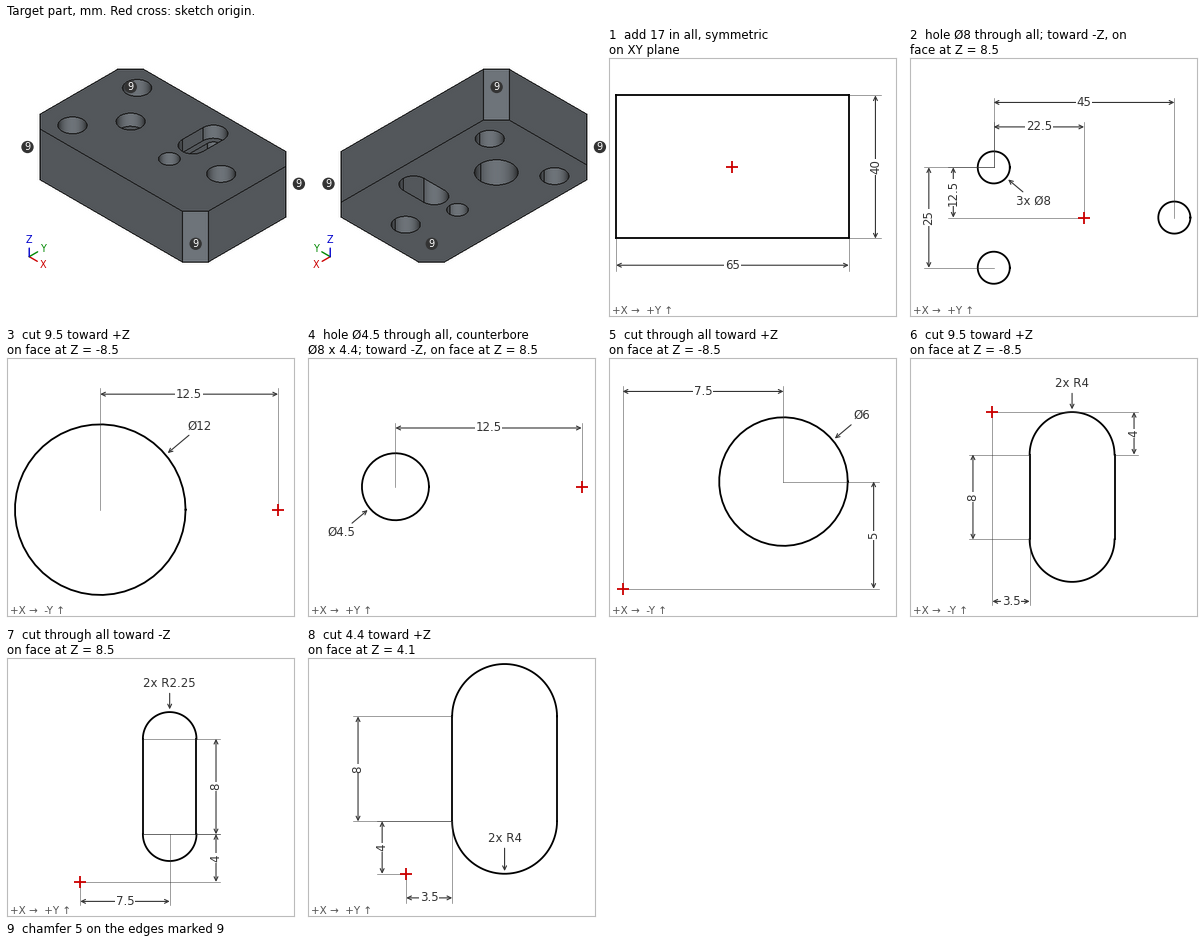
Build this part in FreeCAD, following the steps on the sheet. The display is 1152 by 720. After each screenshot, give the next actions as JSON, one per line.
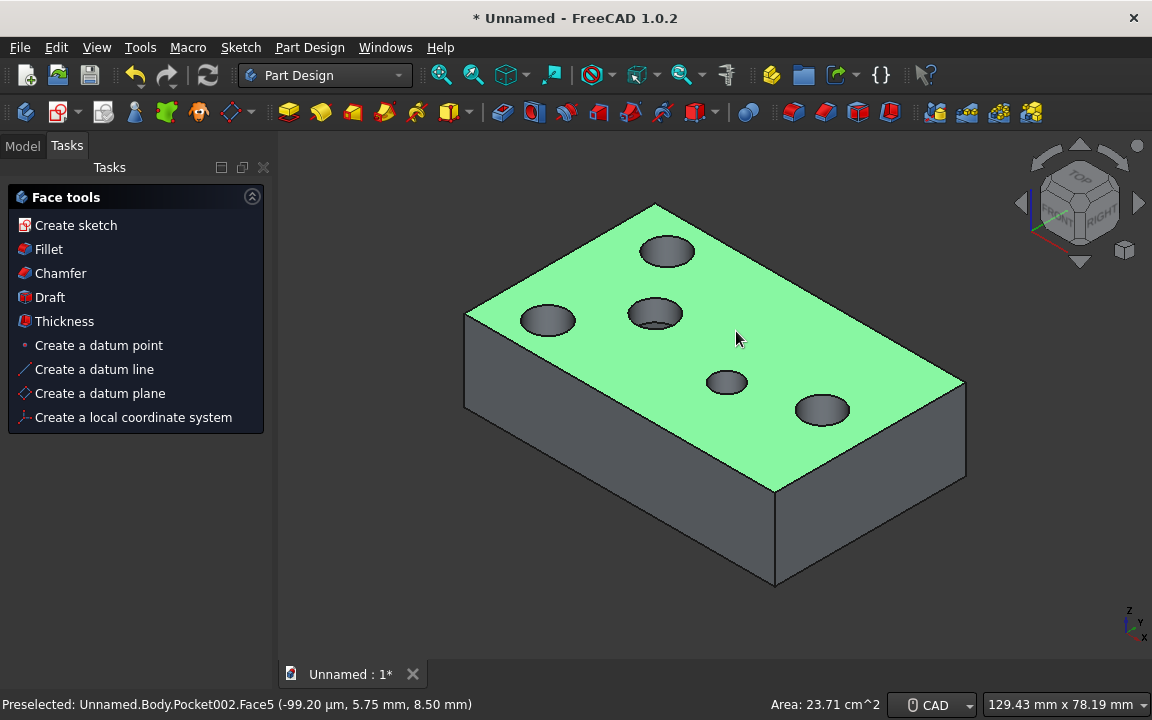
{"action": "left_click", "coordinate": [58, 112]}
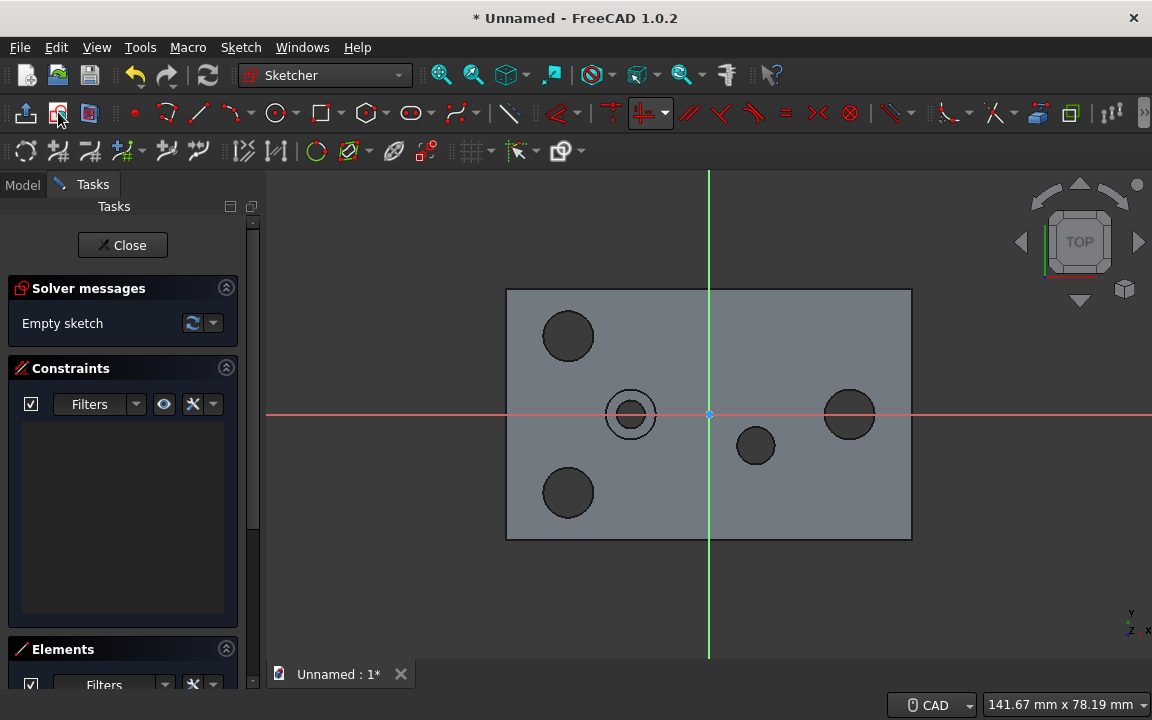
{"action": "scroll", "coordinate": [782, 351], "scroll_direction": "up", "scroll_amount": 6}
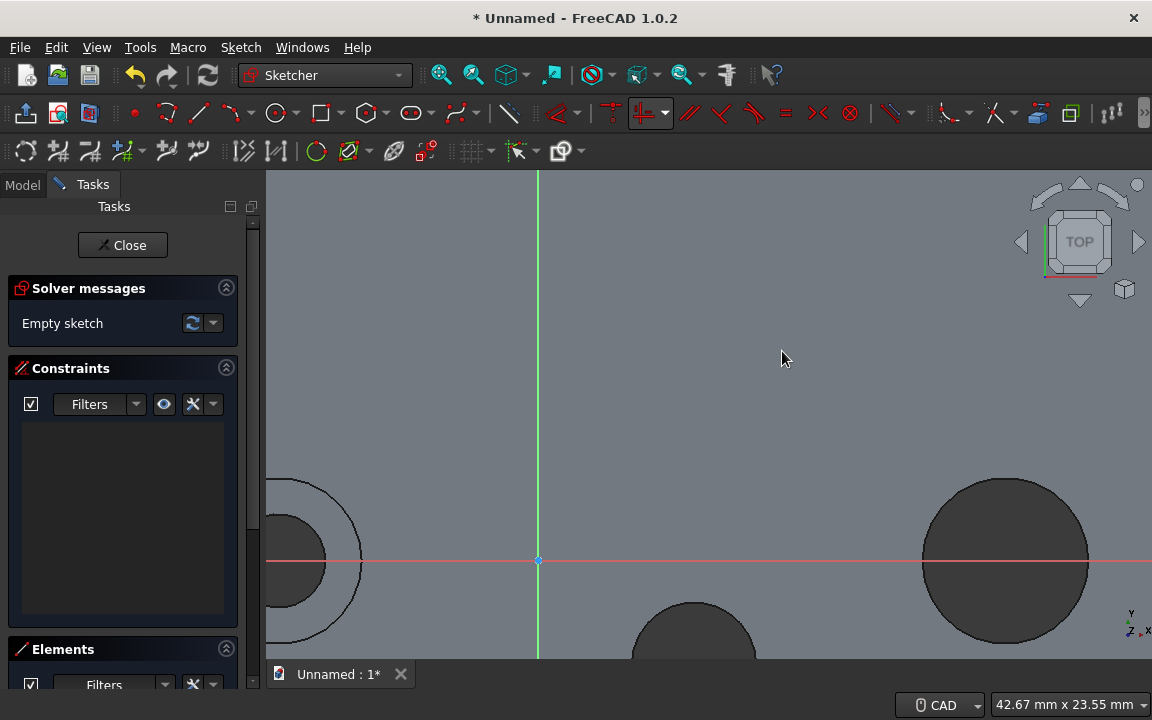
{"action": "key", "text": "g s"}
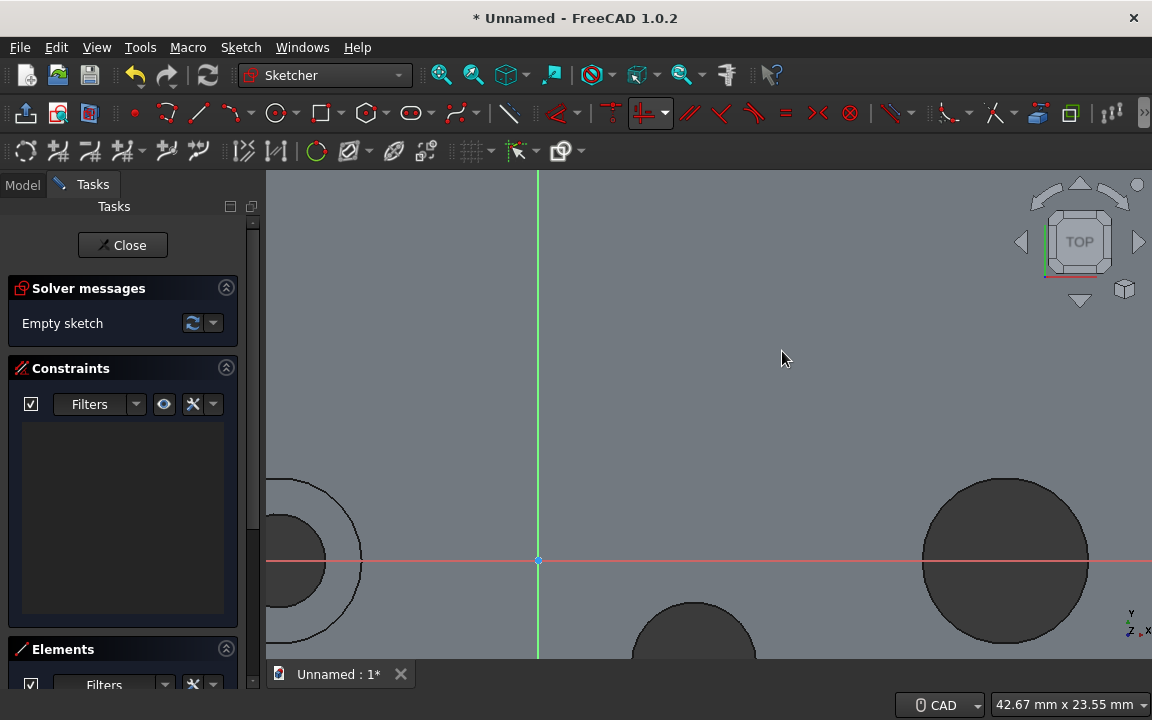
{"action": "left_click", "coordinate": [694, 478]}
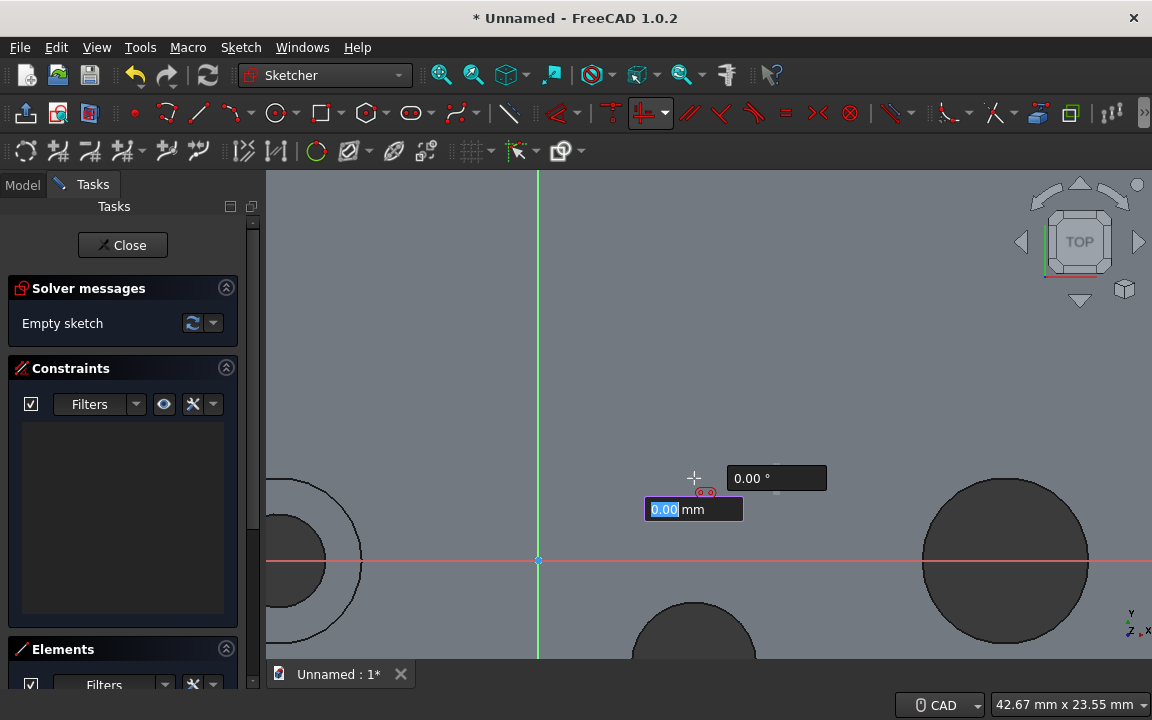
{"action": "left_click", "coordinate": [694, 312]}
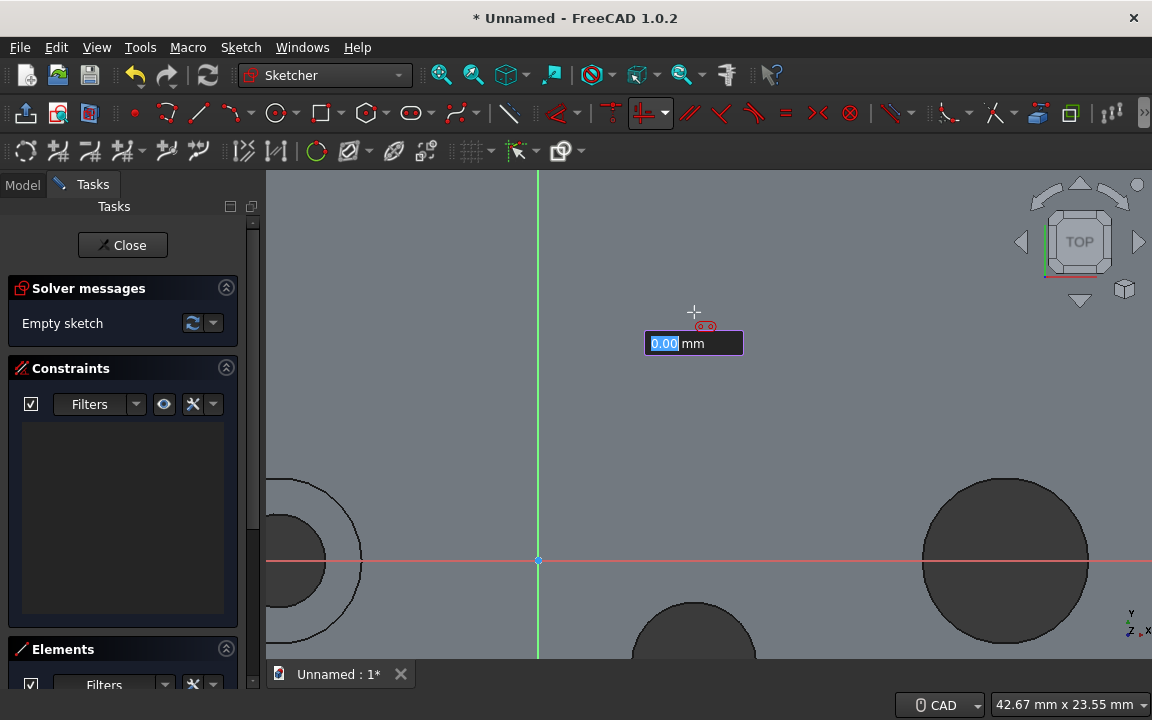
{"action": "left_click", "coordinate": [647, 395]}
{"action": "key", "text": "Escape"}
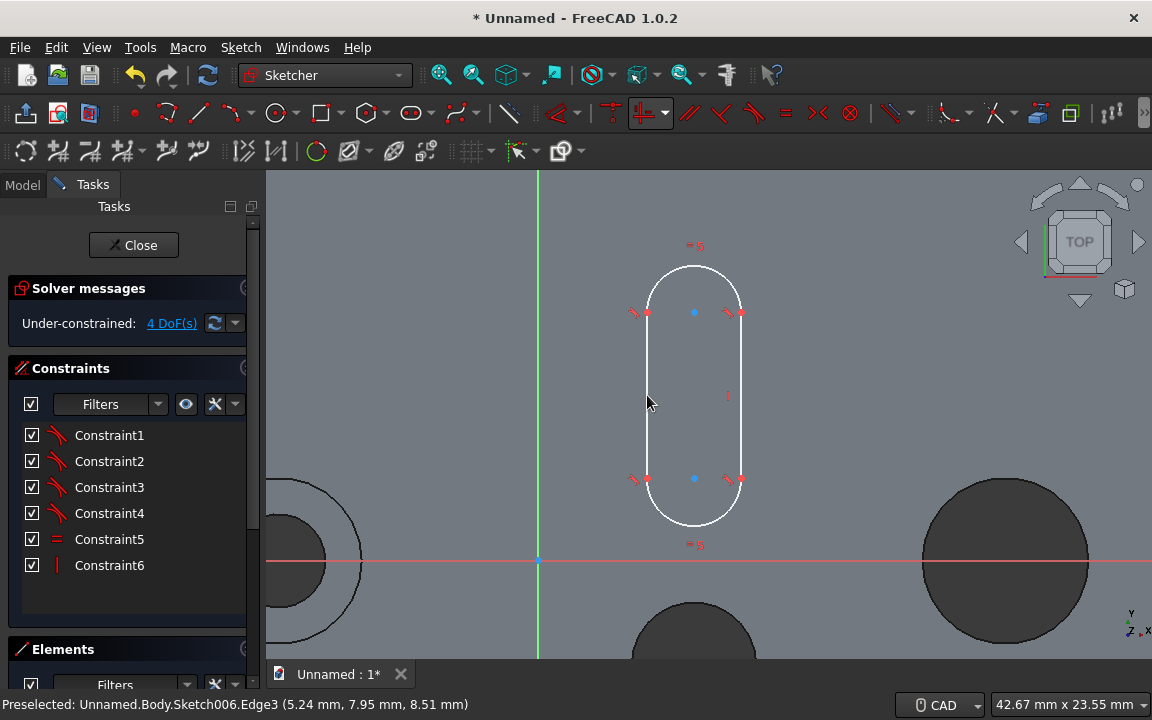
{"action": "left_click", "coordinate": [556, 114]}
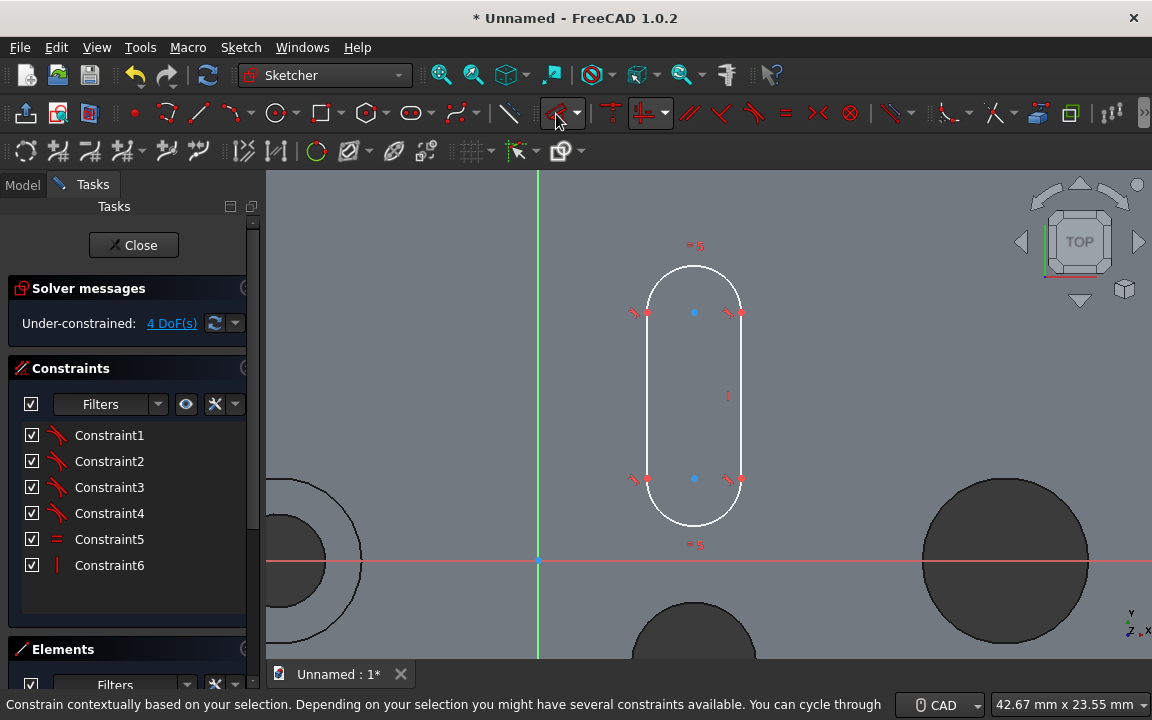
{"action": "left_click", "coordinate": [666, 517]}
{"action": "left_click", "coordinate": [647, 543]}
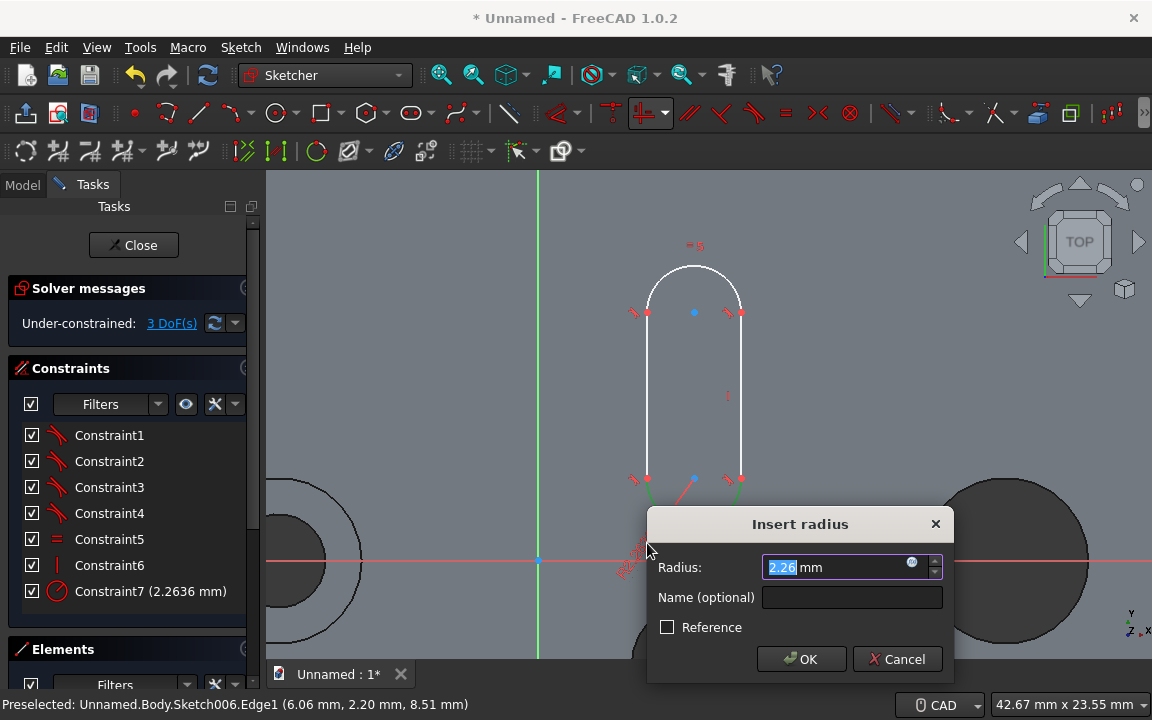
{"action": "type", "text": "2.25"}
{"action": "key", "text": "Return"}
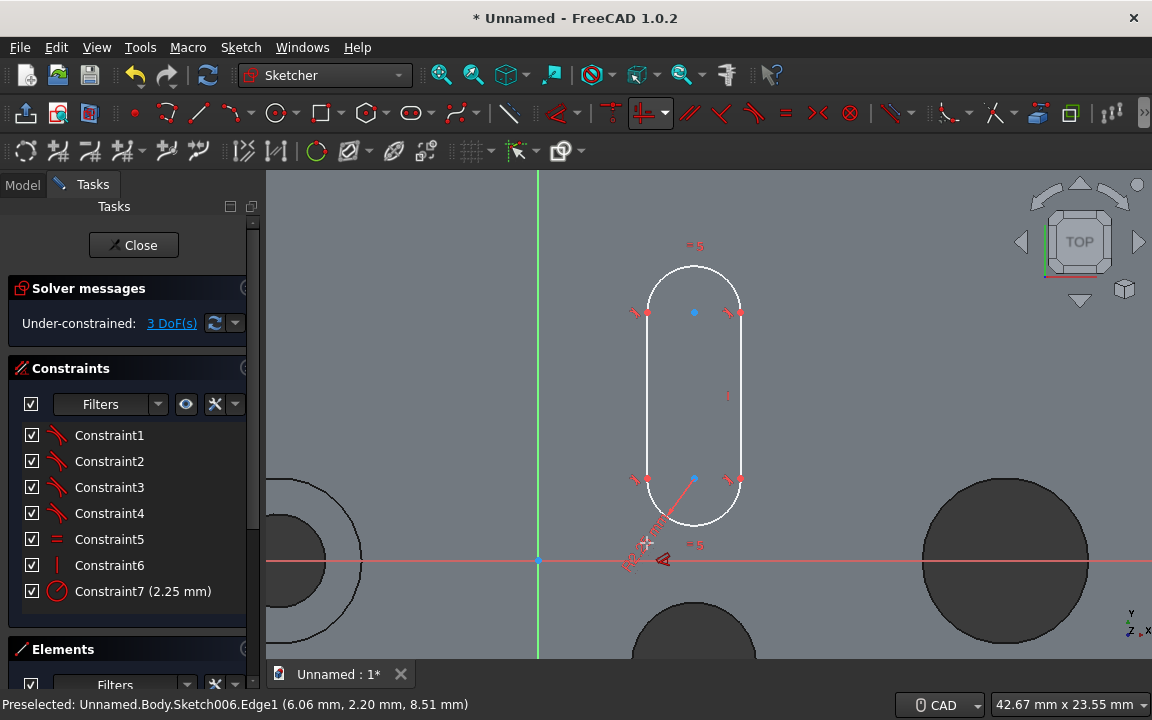
{"action": "left_click", "coordinate": [647, 429]}
{"action": "left_click", "coordinate": [681, 396]}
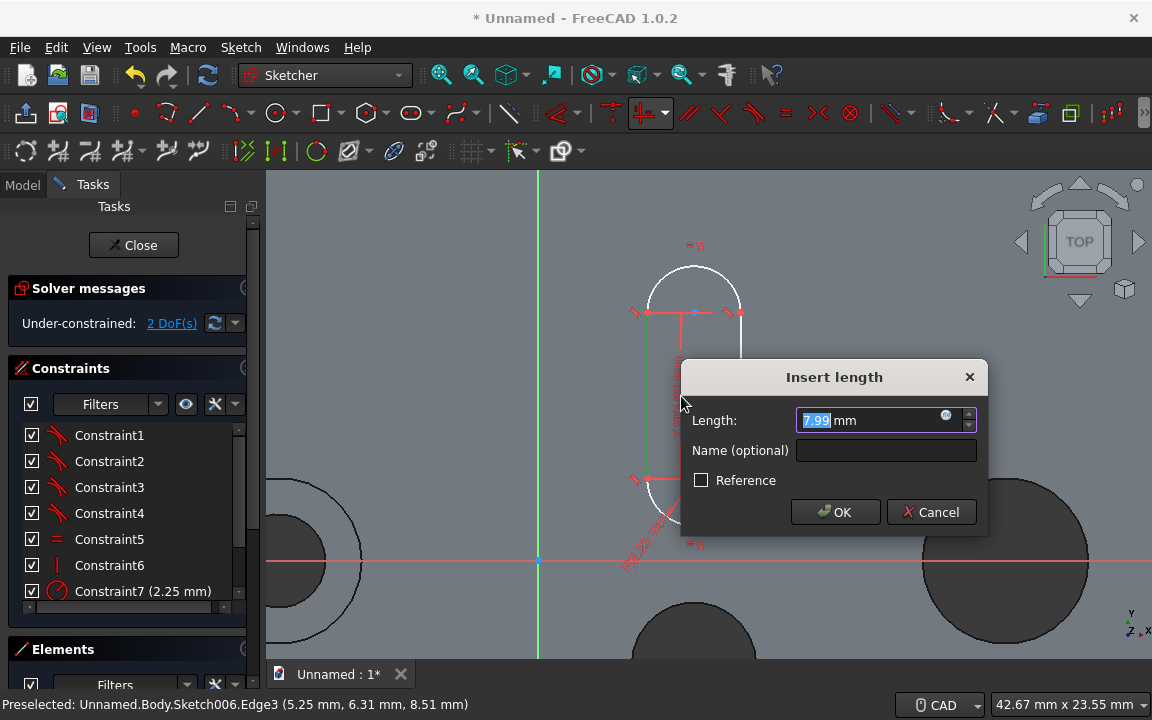
{"action": "type", "text": "8"}
{"action": "key", "text": "Return"}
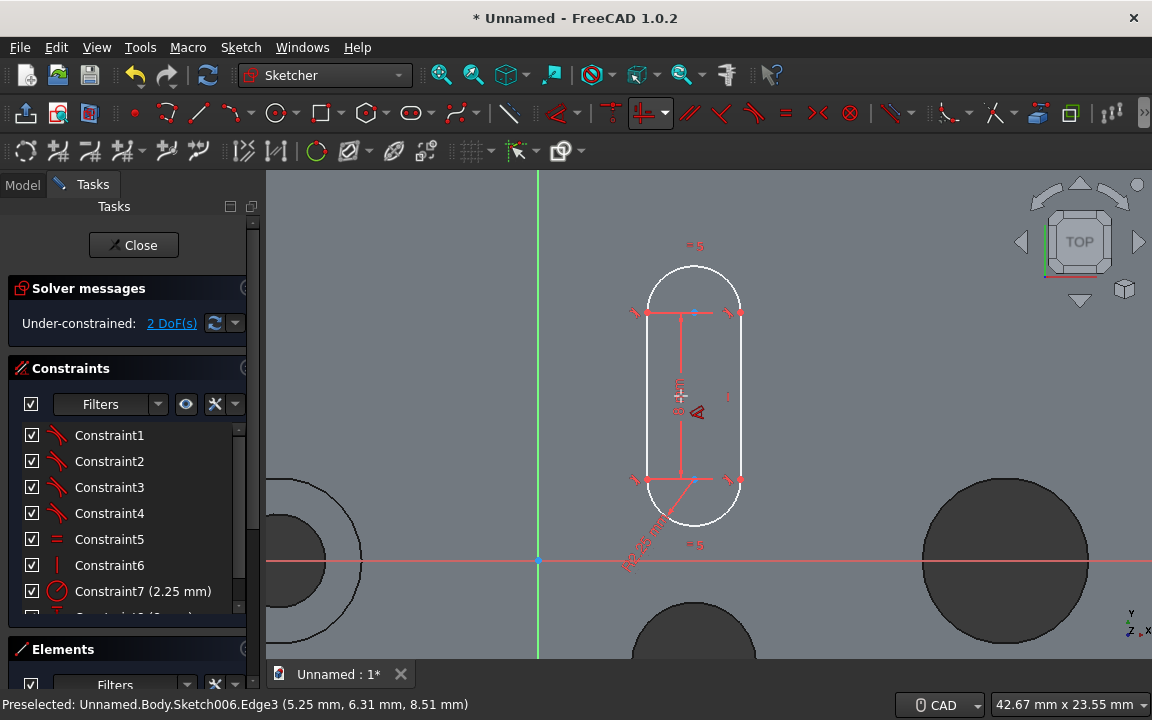
{"action": "left_click", "coordinate": [647, 479]}
{"action": "left_click", "coordinate": [504, 520]}